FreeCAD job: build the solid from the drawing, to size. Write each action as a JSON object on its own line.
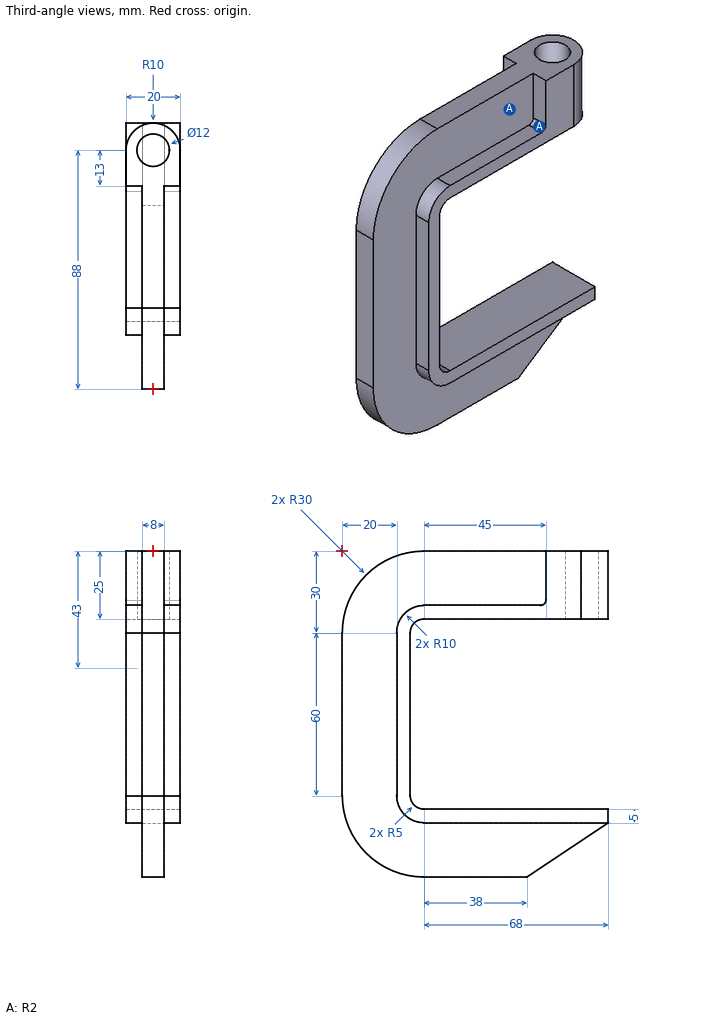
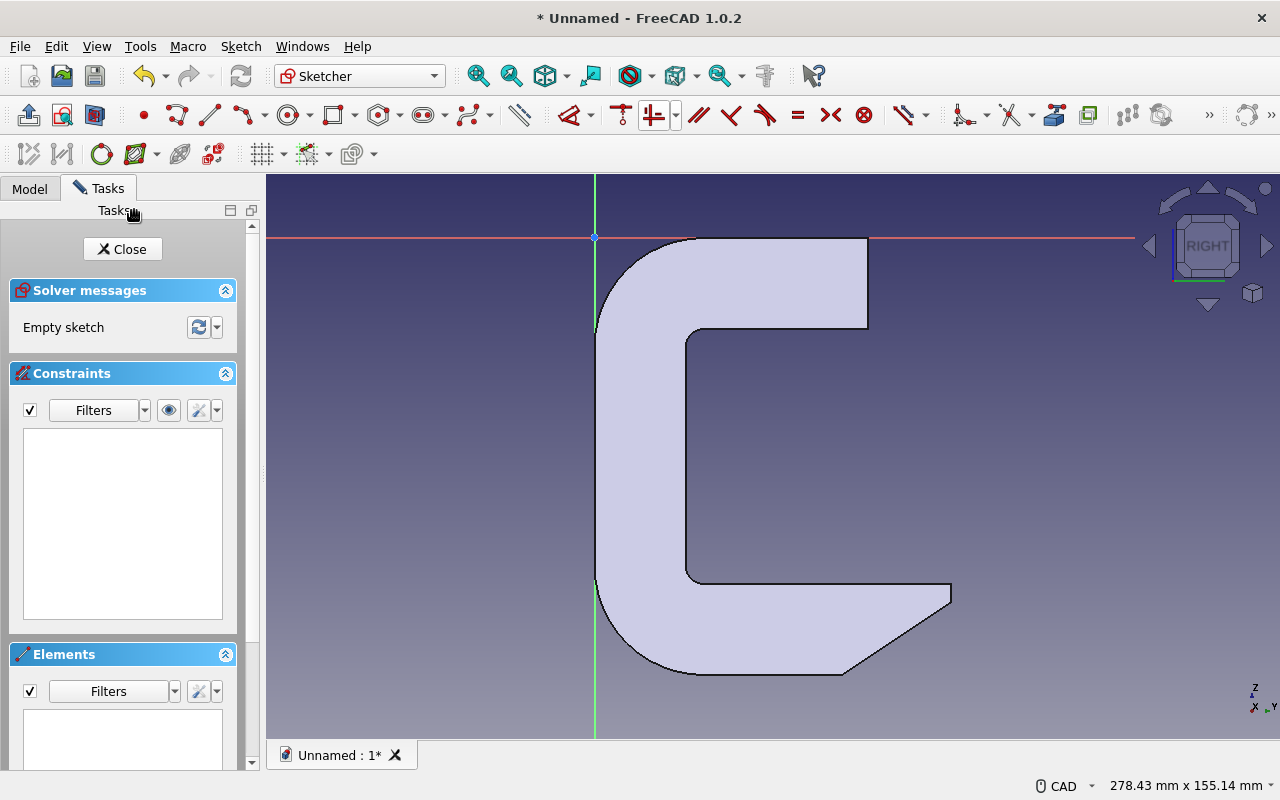
{"action": "left_click", "coordinate": [95, 116]}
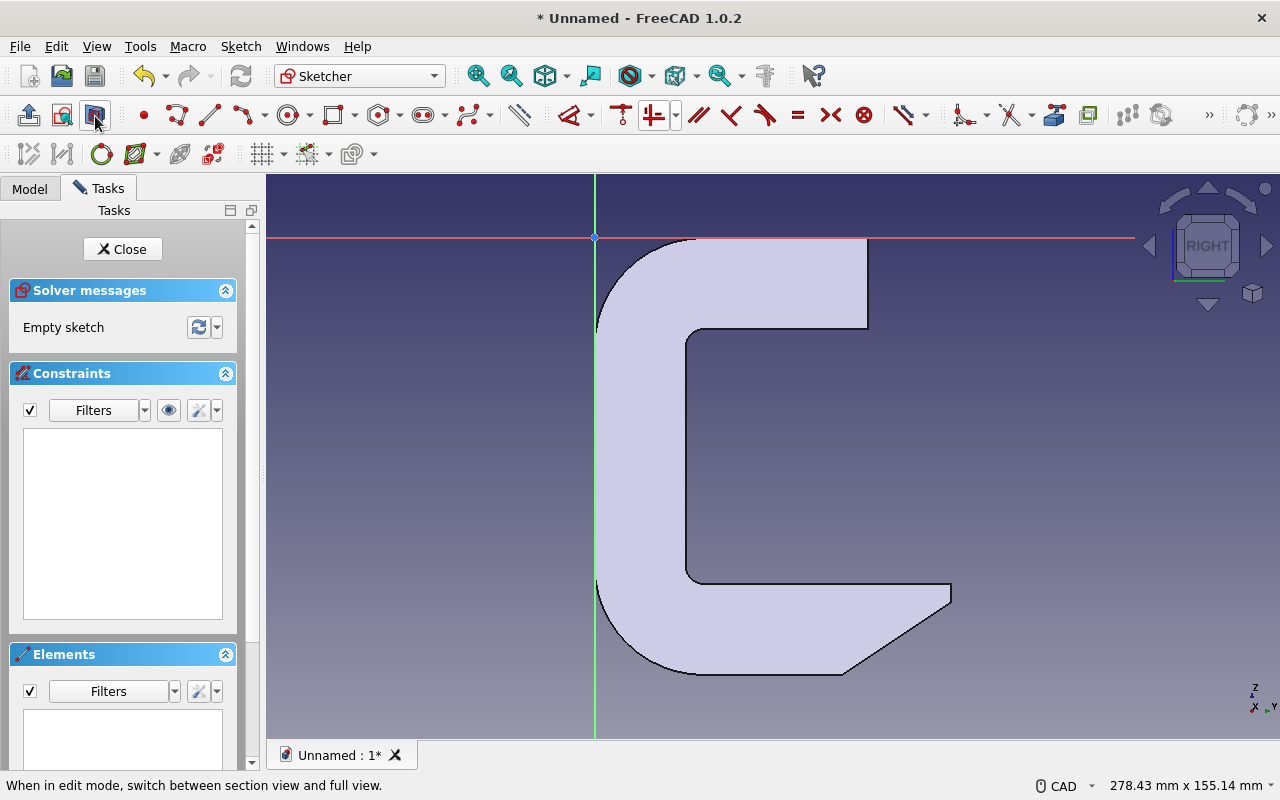
{"action": "key", "text": "g l"}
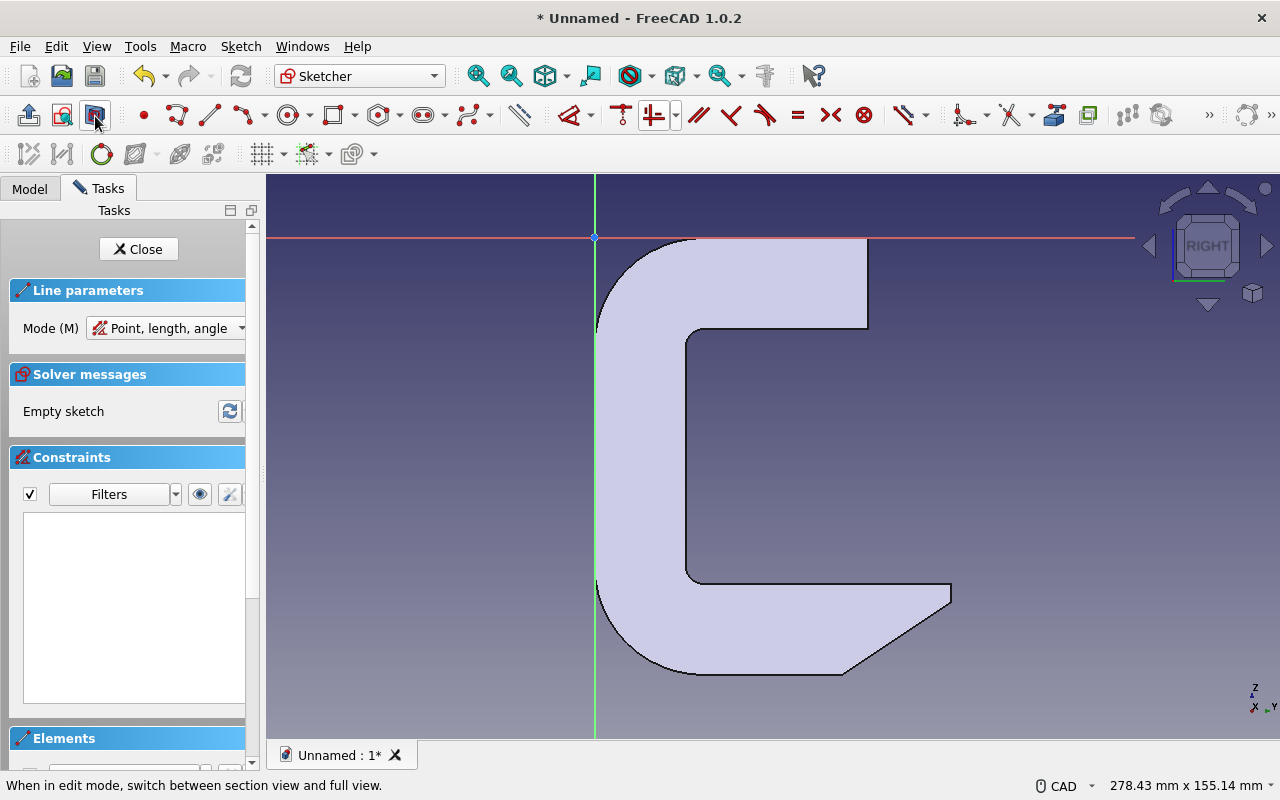
{"action": "left_click", "coordinate": [667, 347]}
{"action": "left_click", "coordinate": [667, 566]}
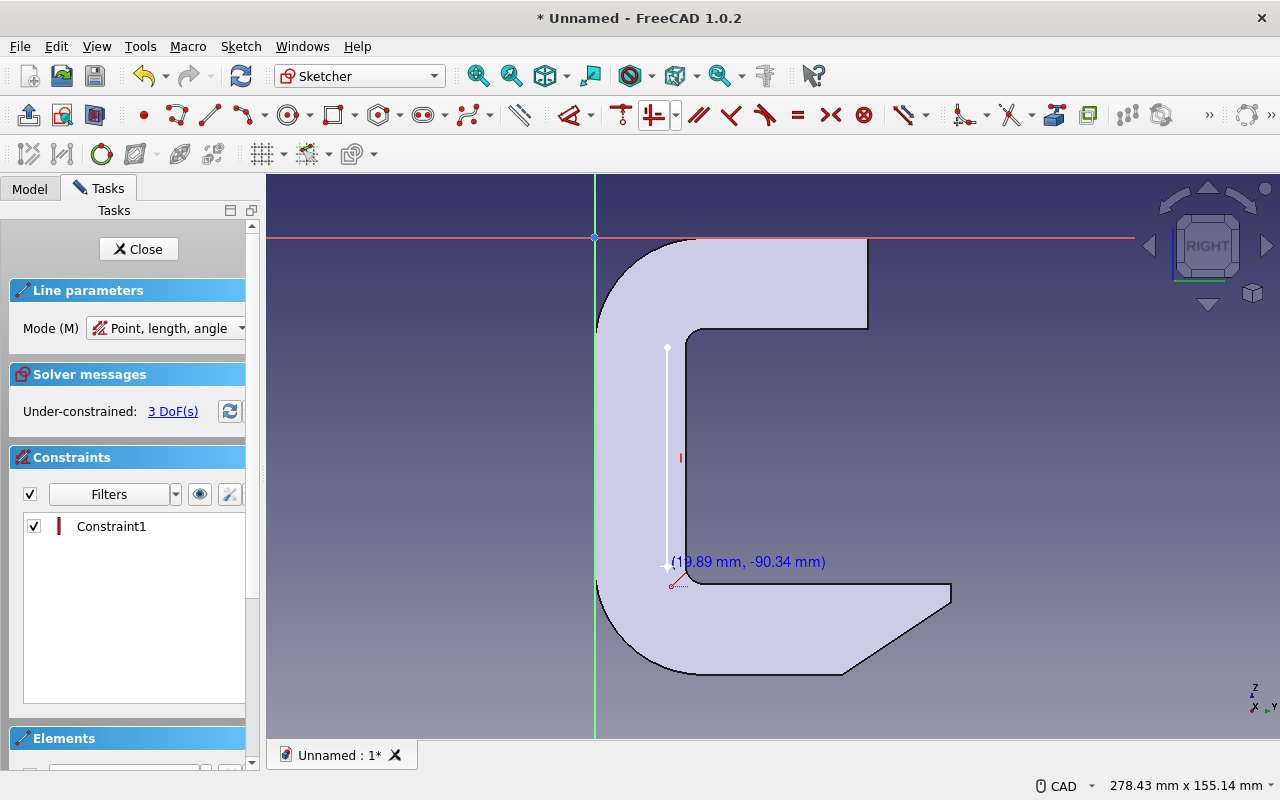
{"action": "key", "text": "g m"}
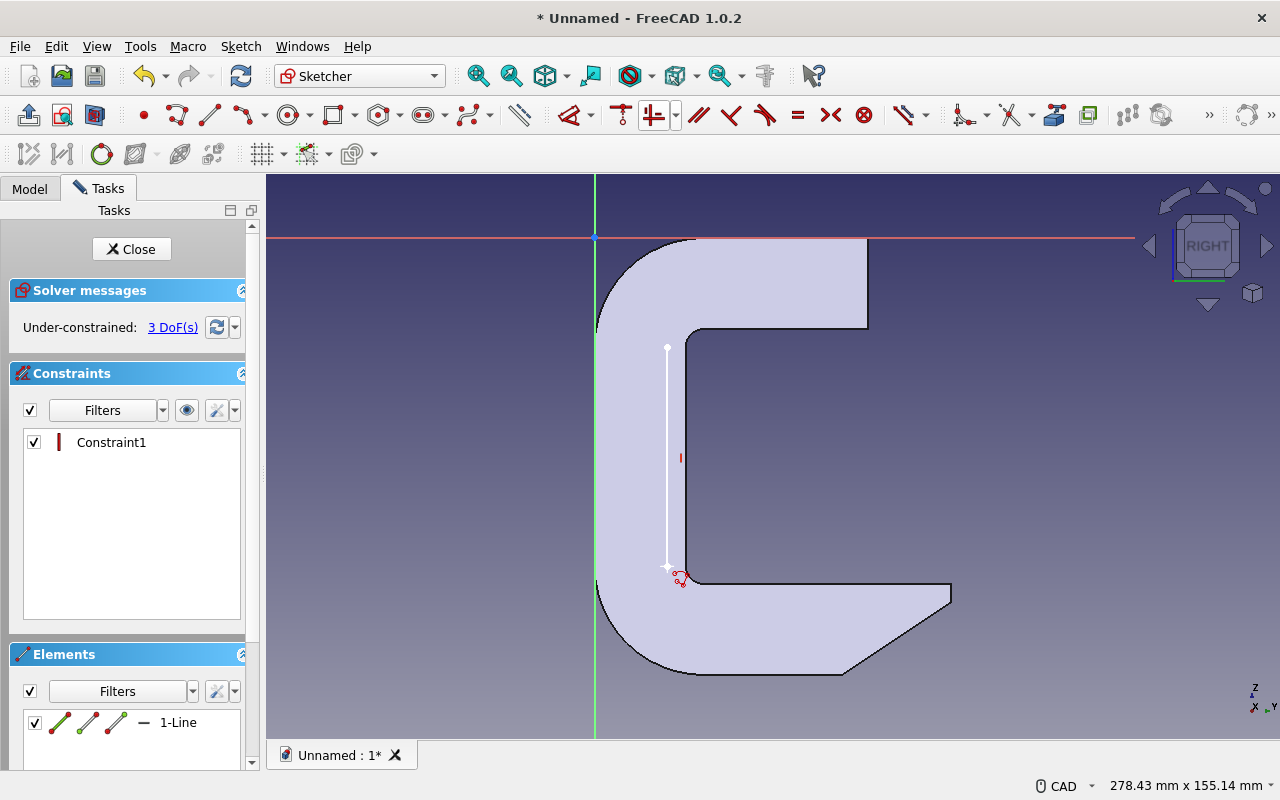
{"action": "left_click", "coordinate": [704, 602]}
{"action": "left_click", "coordinate": [951, 602]}
{"action": "left_click", "coordinate": [951, 584]}
{"action": "left_click", "coordinate": [704, 584]}
{"action": "right_click", "coordinate": [704, 584]}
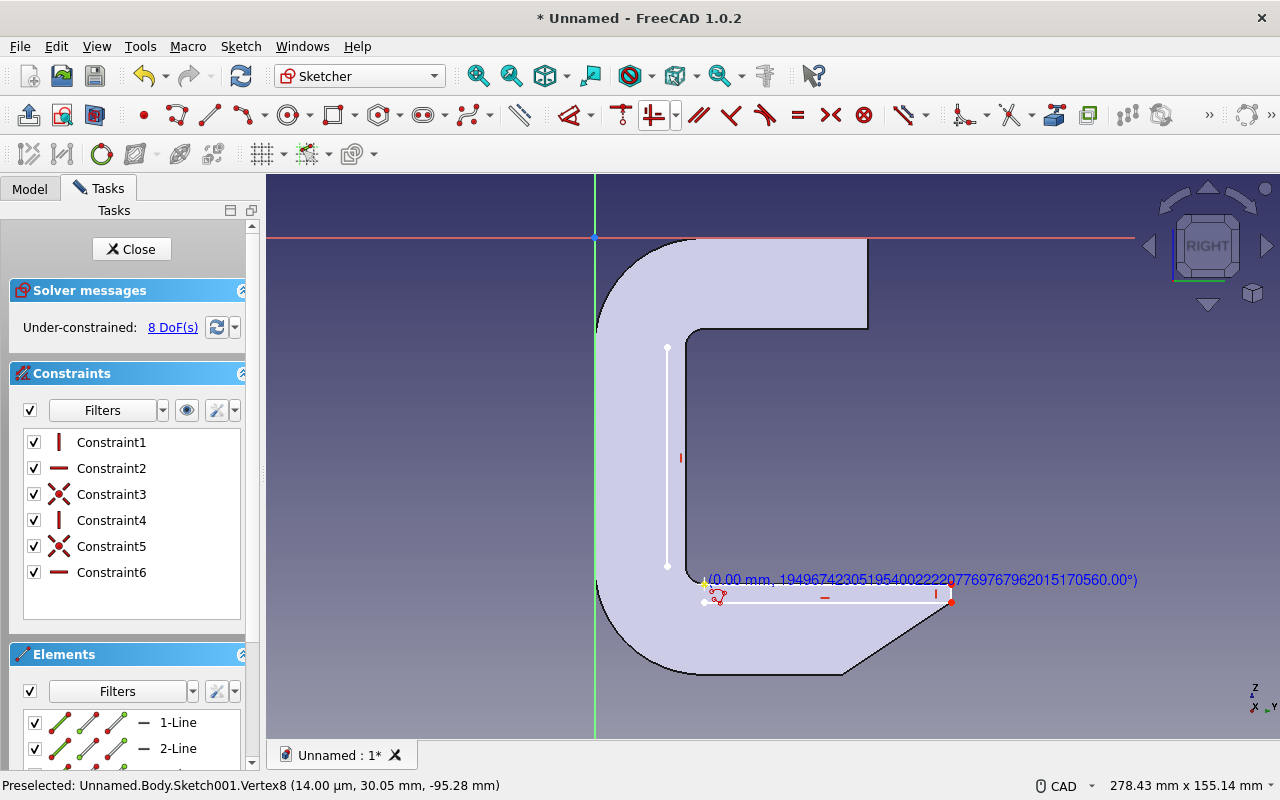
{"action": "left_click", "coordinate": [210, 116]}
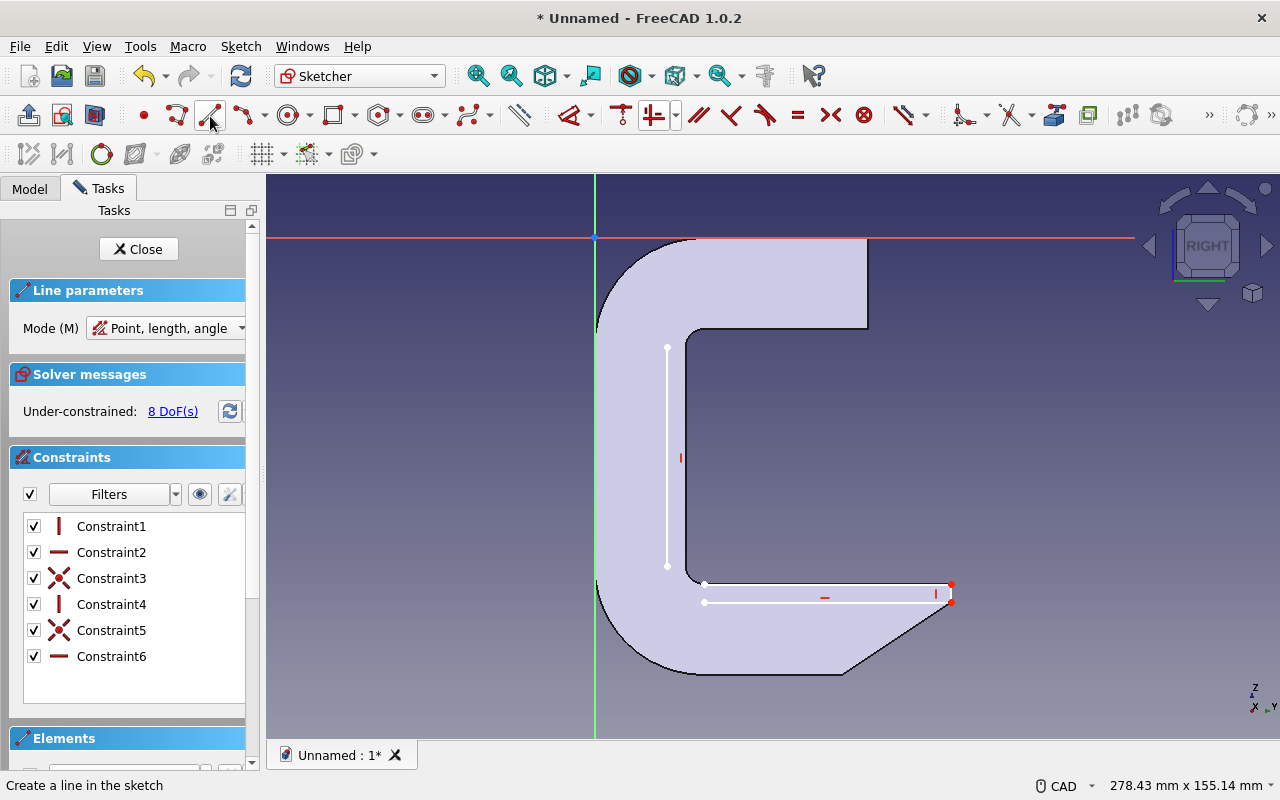
{"action": "left_click", "coordinate": [686, 566]}
{"action": "left_click", "coordinate": [686, 347]}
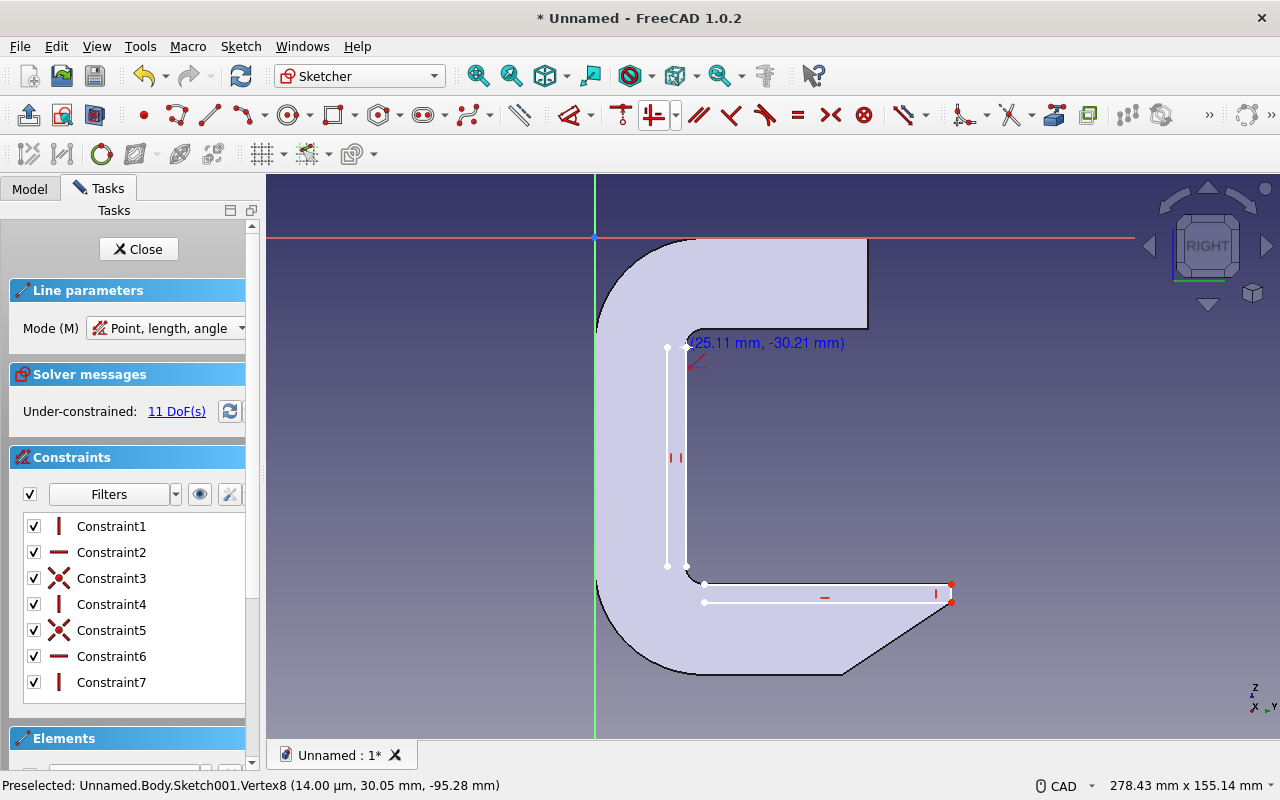
{"action": "key", "text": "g m"}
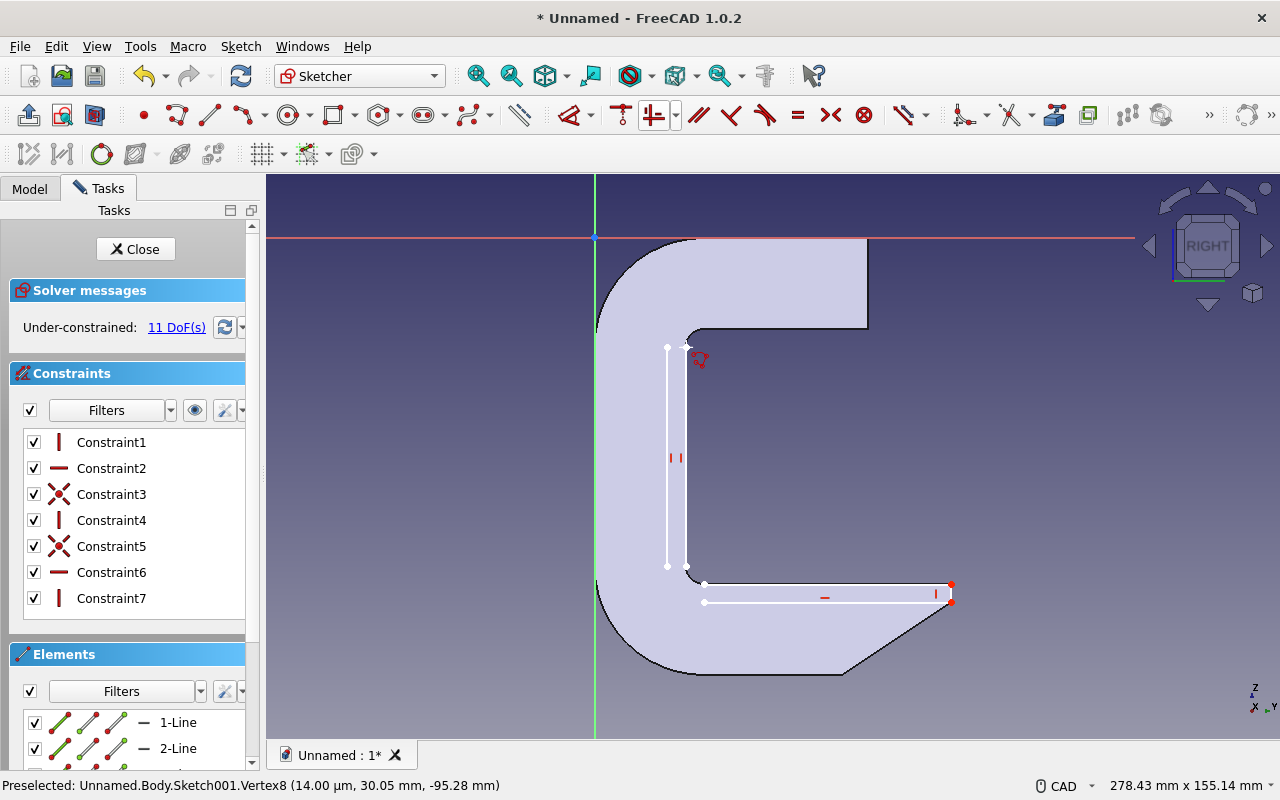
{"action": "left_click", "coordinate": [704, 329]}
{"action": "left_click", "coordinate": [868, 329]}
{"action": "left_click", "coordinate": [868, 311]}
{"action": "left_click", "coordinate": [704, 311]}
{"action": "right_click", "coordinate": [704, 311]}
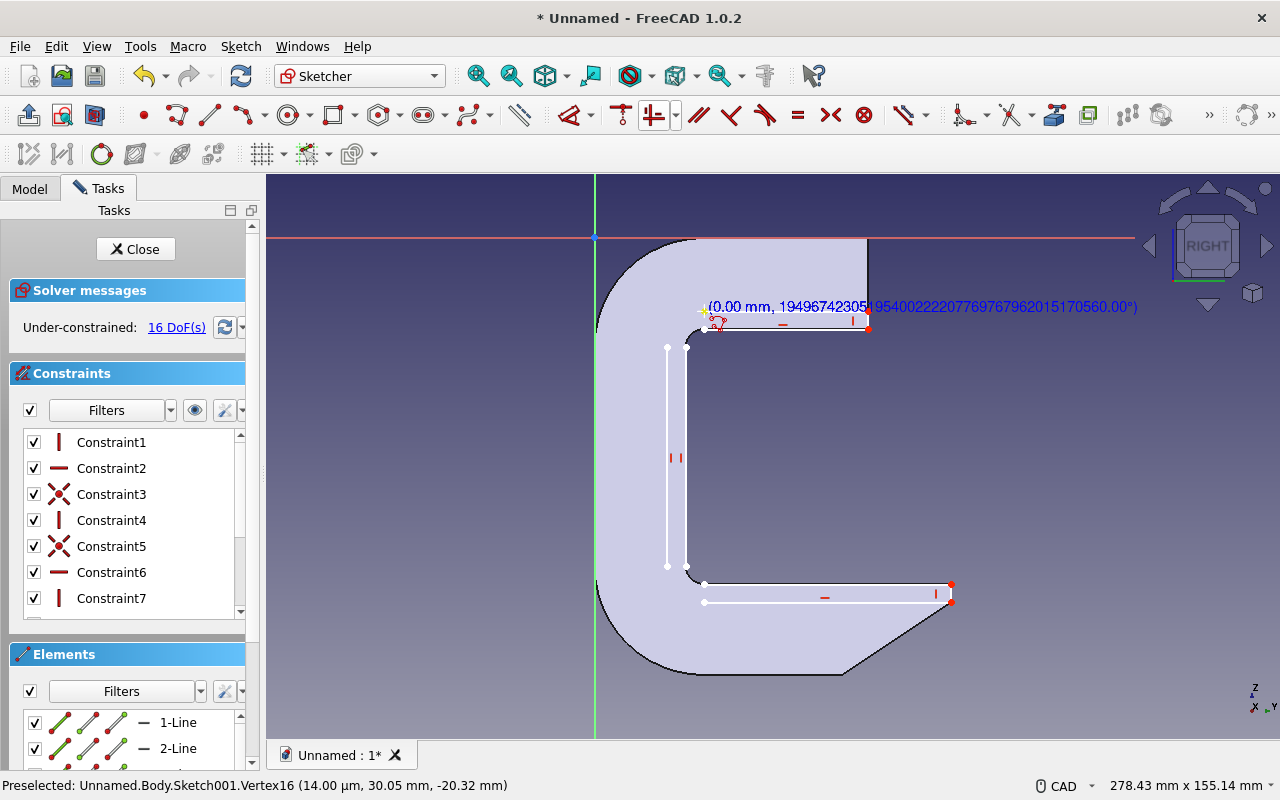
{"action": "key", "text": "g 3 a"}